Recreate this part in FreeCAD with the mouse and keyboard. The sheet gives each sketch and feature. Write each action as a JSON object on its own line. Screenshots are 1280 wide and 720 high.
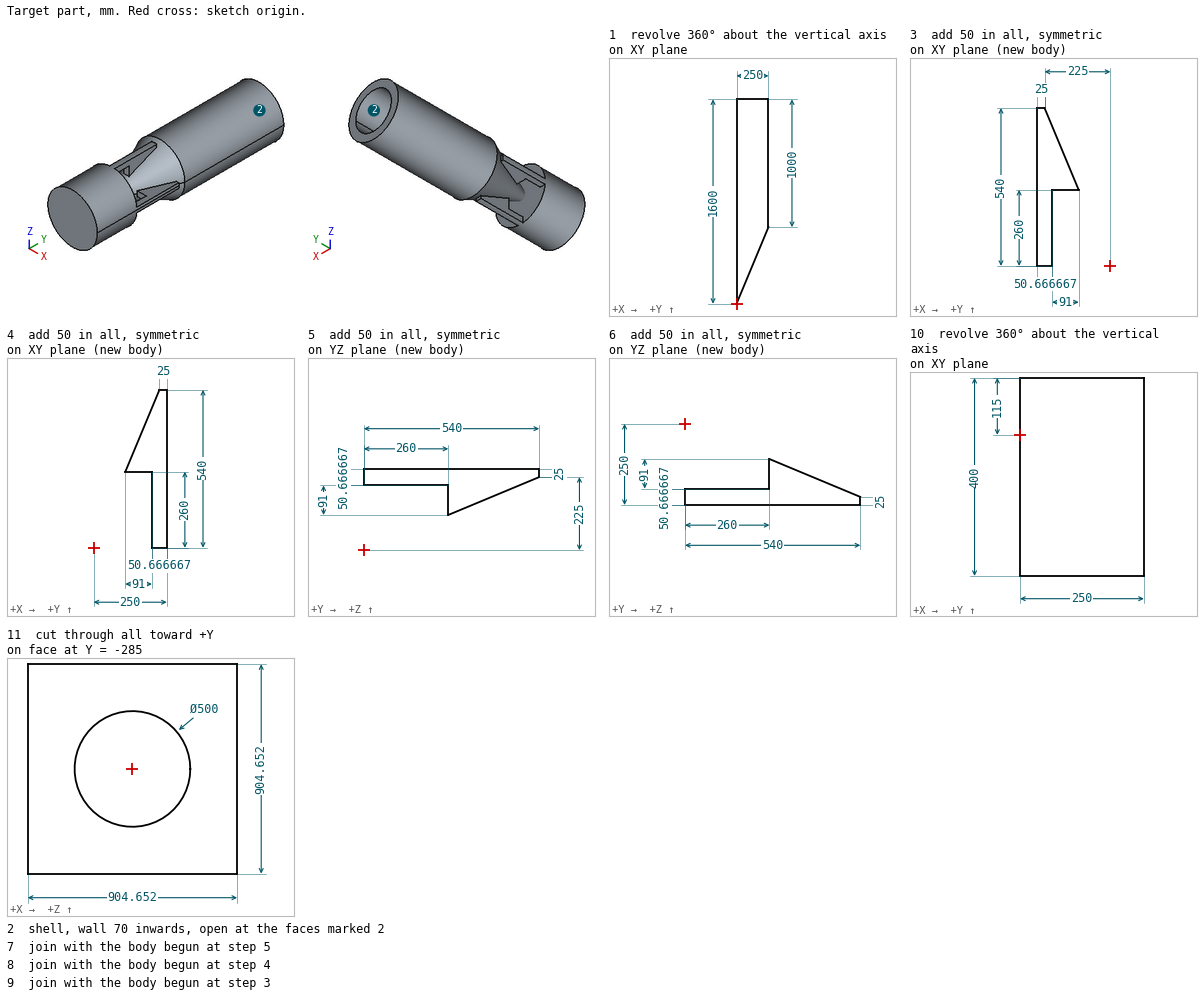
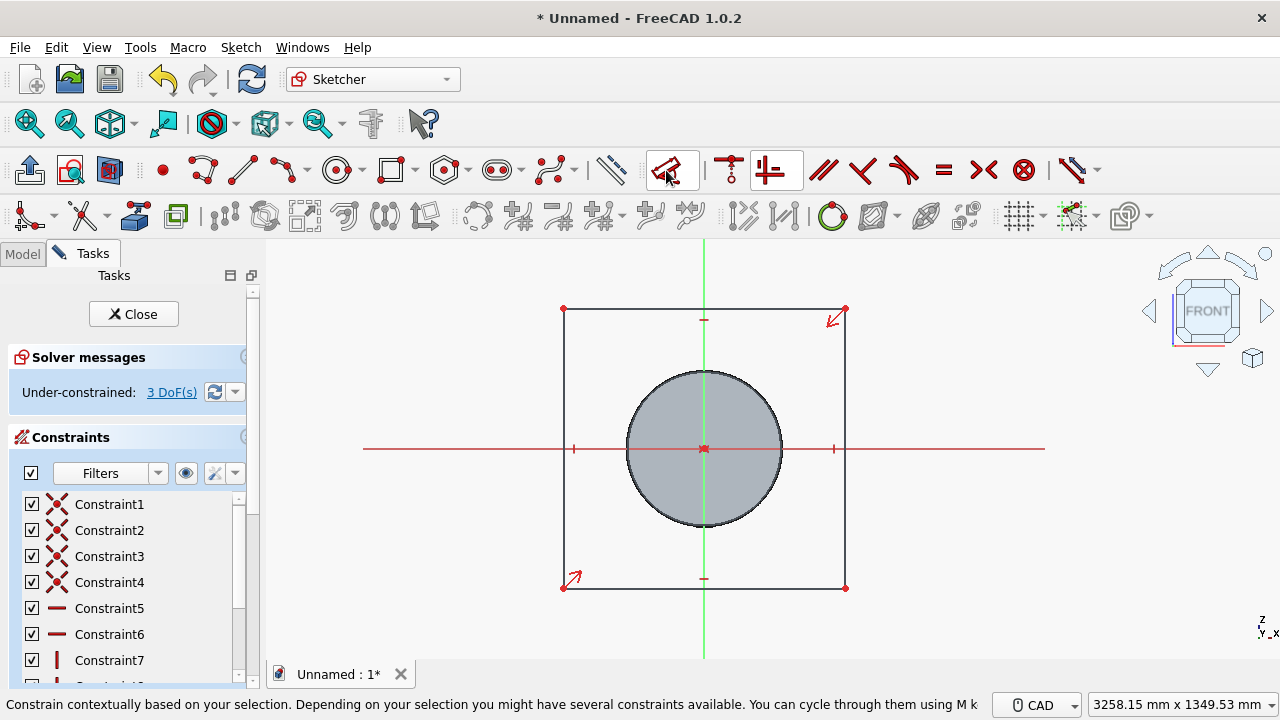
{"action": "left_click", "coordinate": [758, 394]}
{"action": "left_click", "coordinate": [780, 371]}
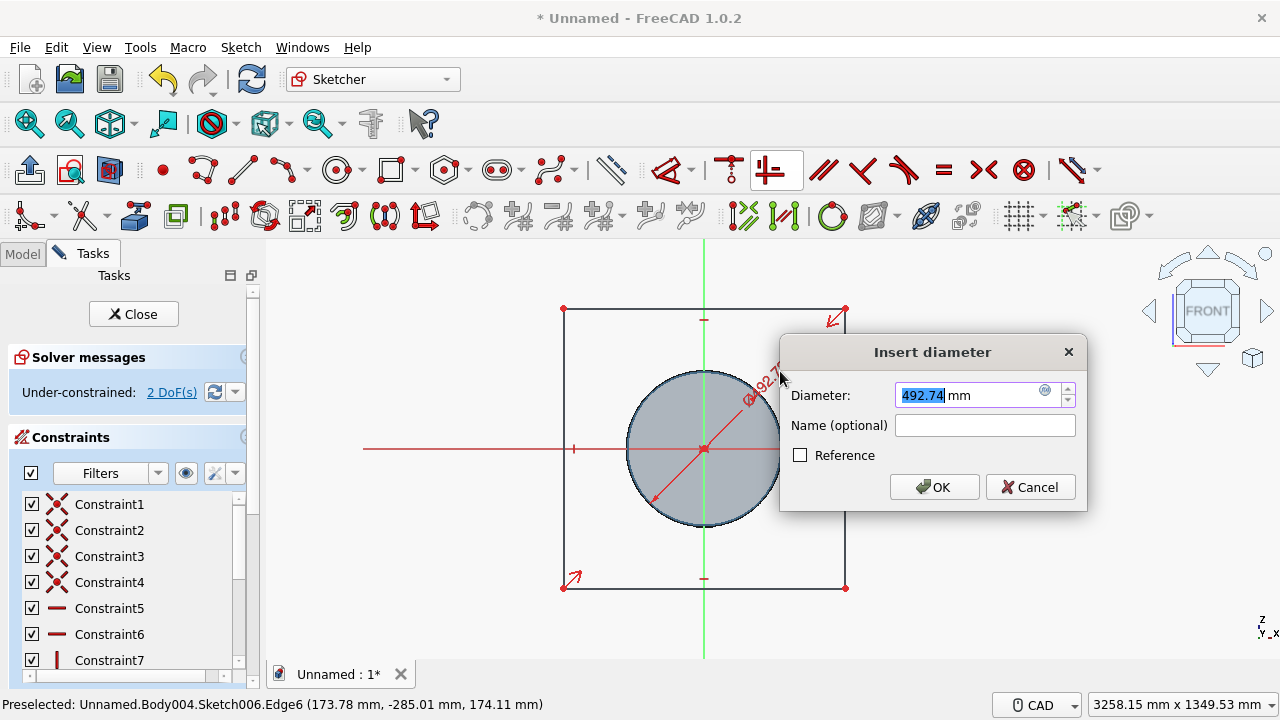
{"action": "type", "text": "500"}
{"action": "key", "text": "Return"}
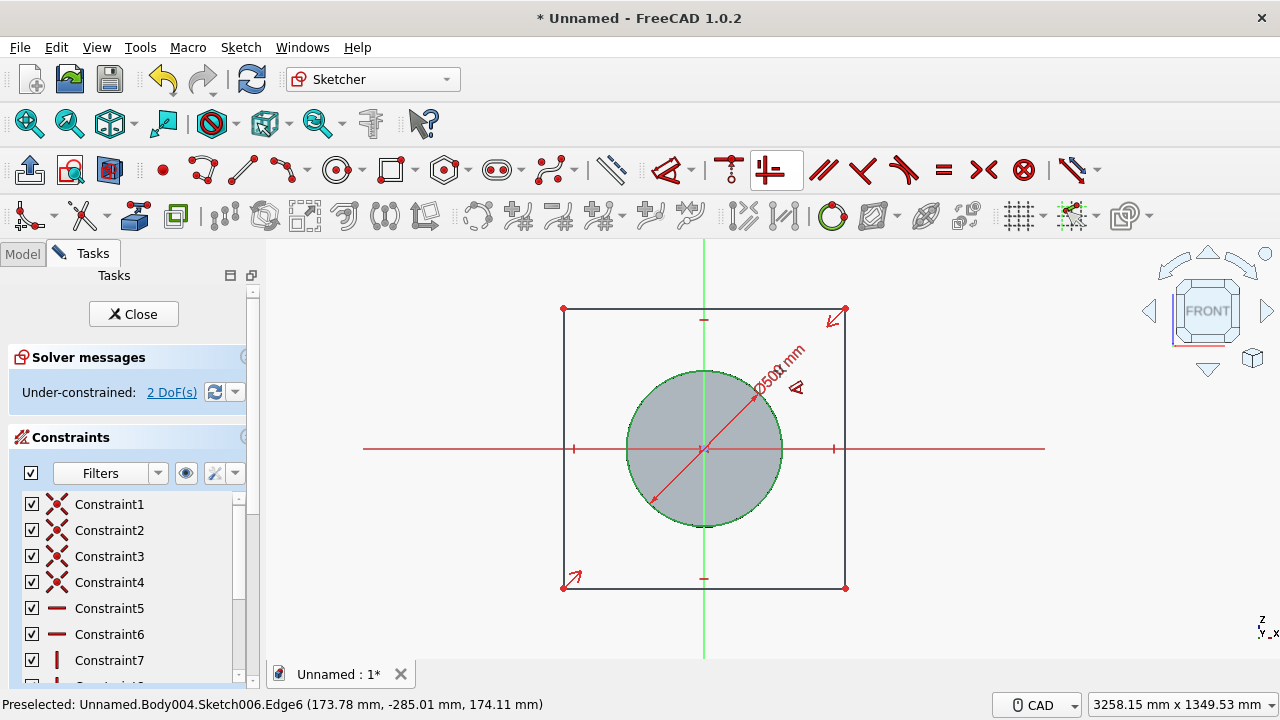
{"action": "left_click", "coordinate": [648, 589]}
{"action": "left_click", "coordinate": [640, 623]}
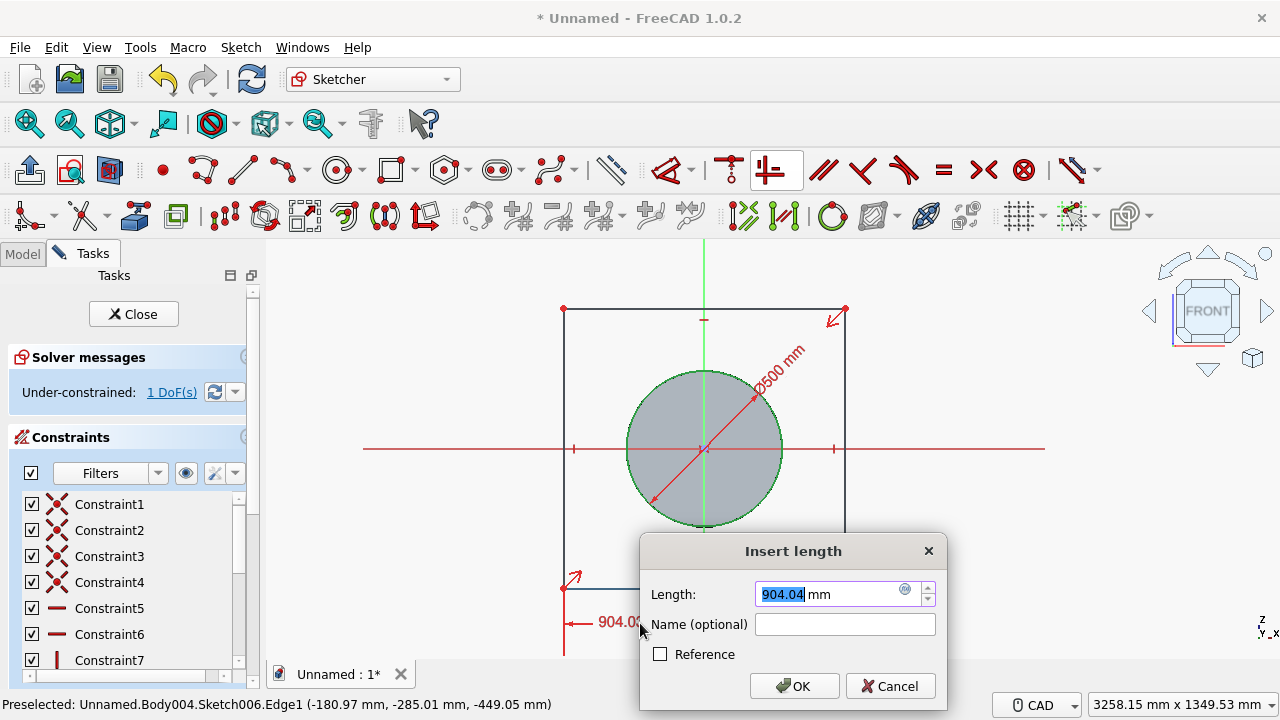
{"action": "type", "text": "904.652"}
{"action": "key", "text": "Return"}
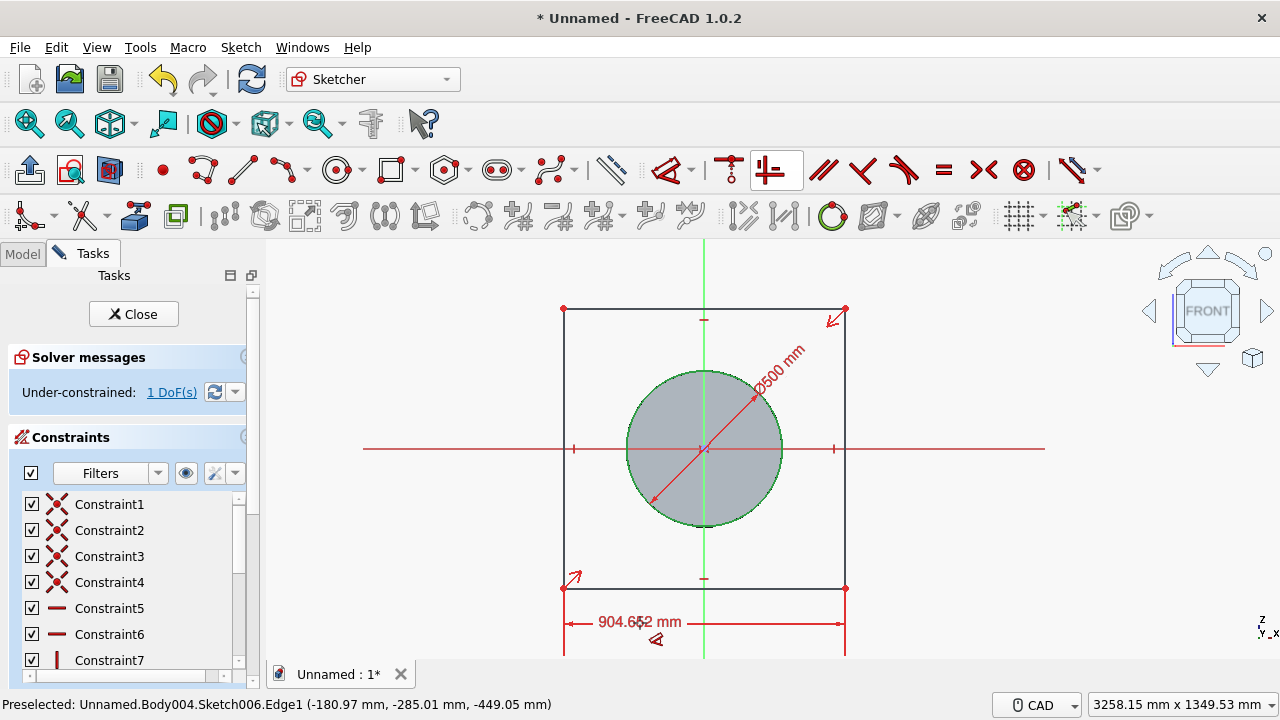
{"action": "left_click", "coordinate": [845, 505]}
{"action": "left_click", "coordinate": [879, 384]}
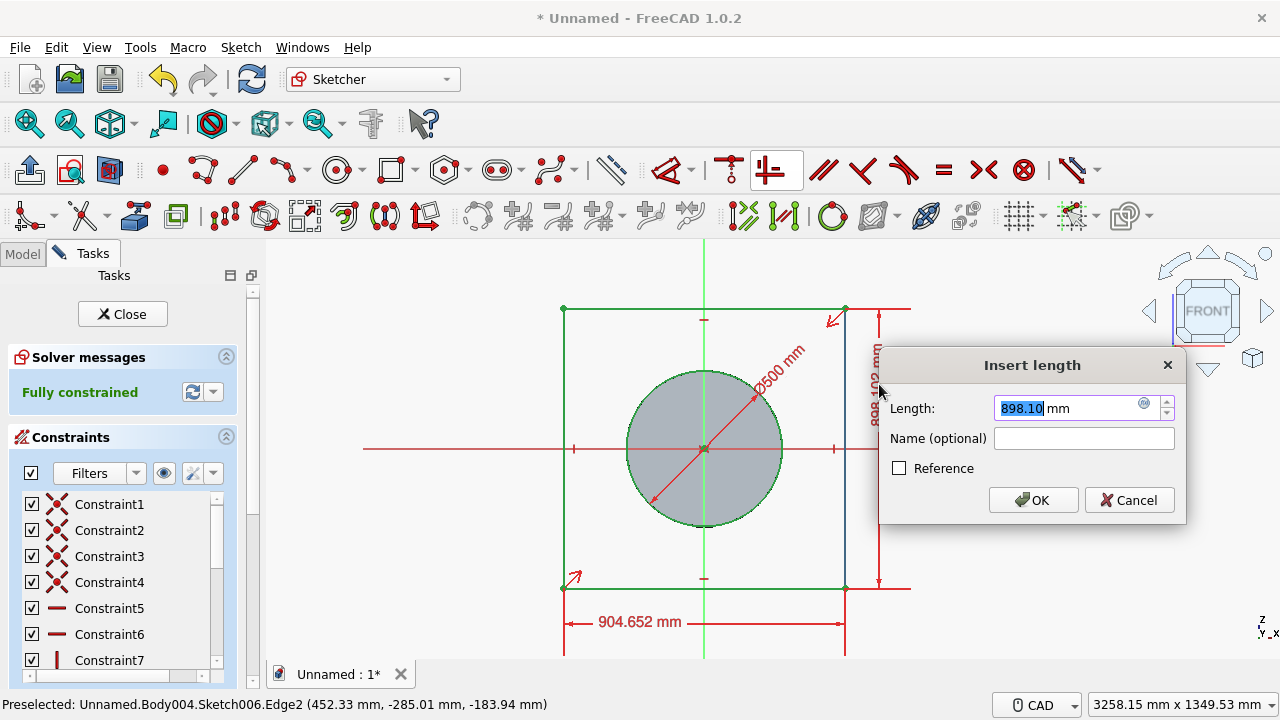
{"action": "type", "text": "904.652"}
{"action": "key", "text": "Return"}
{"action": "key", "text": "Escape"}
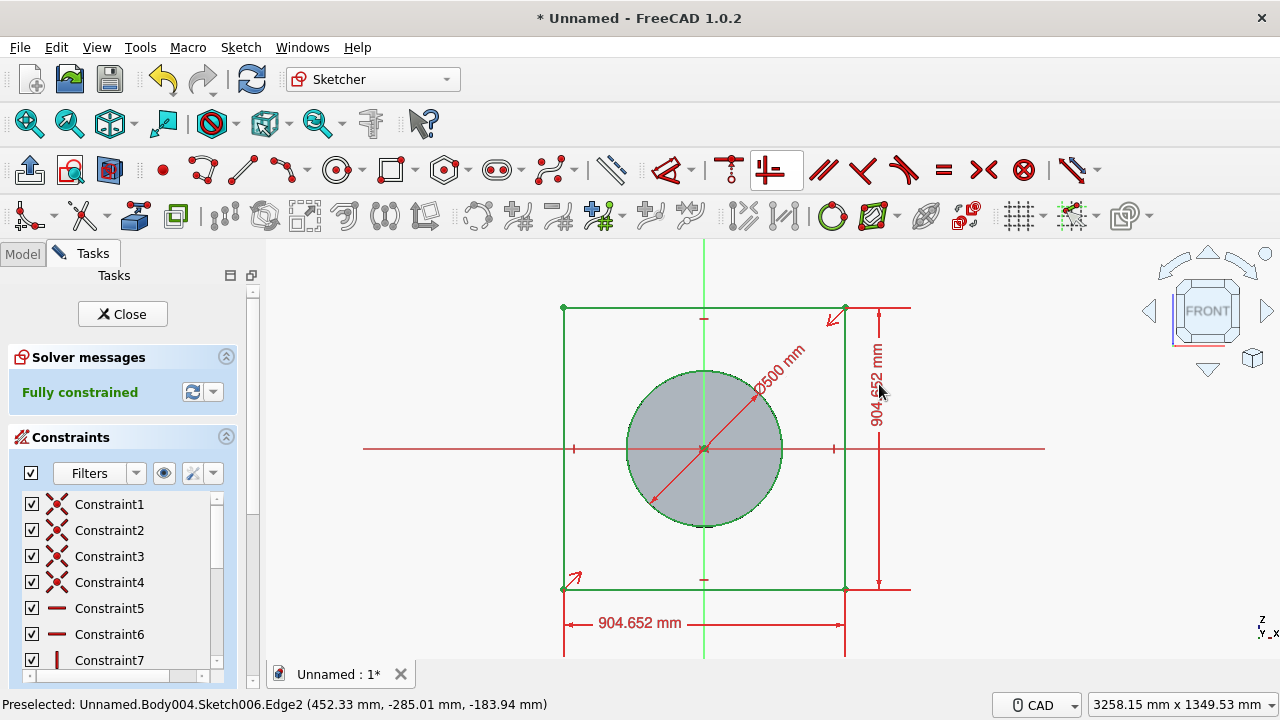
{"action": "left_click", "coordinate": [123, 314]}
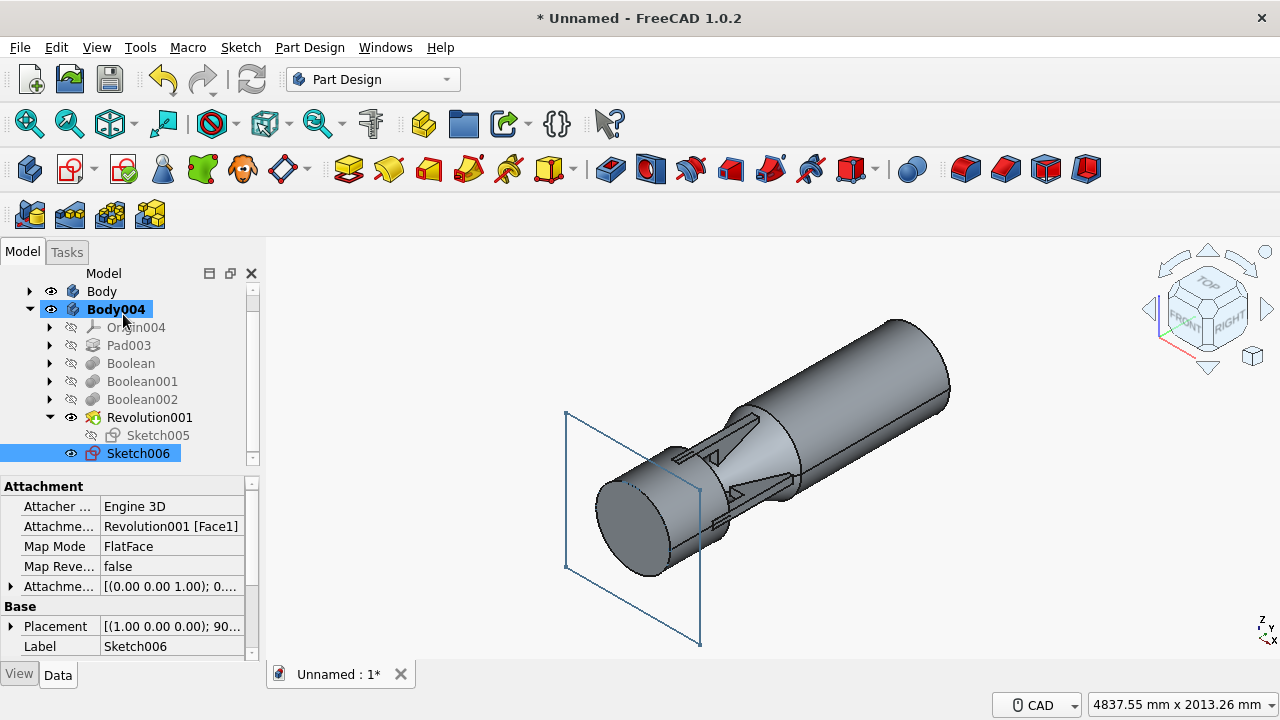
{"action": "left_click", "coordinate": [612, 170]}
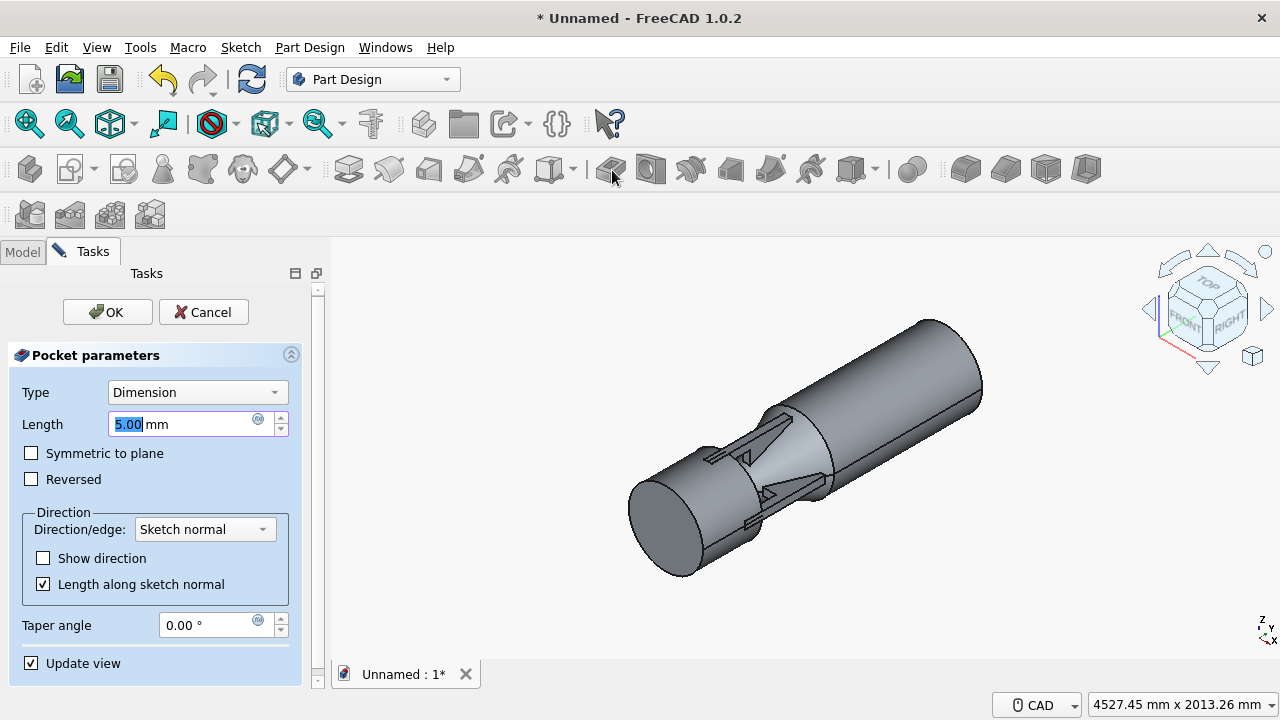
{"action": "left_click", "coordinate": [198, 392]}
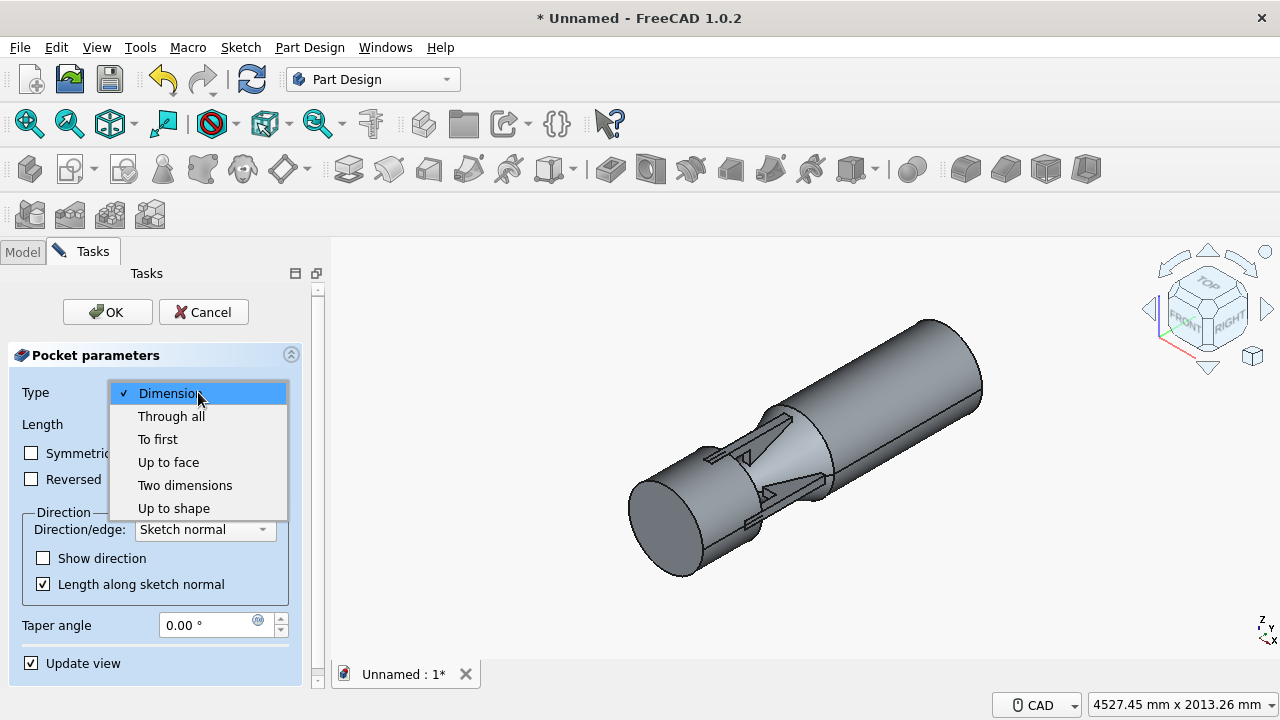
{"action": "left_click", "coordinate": [198, 416]}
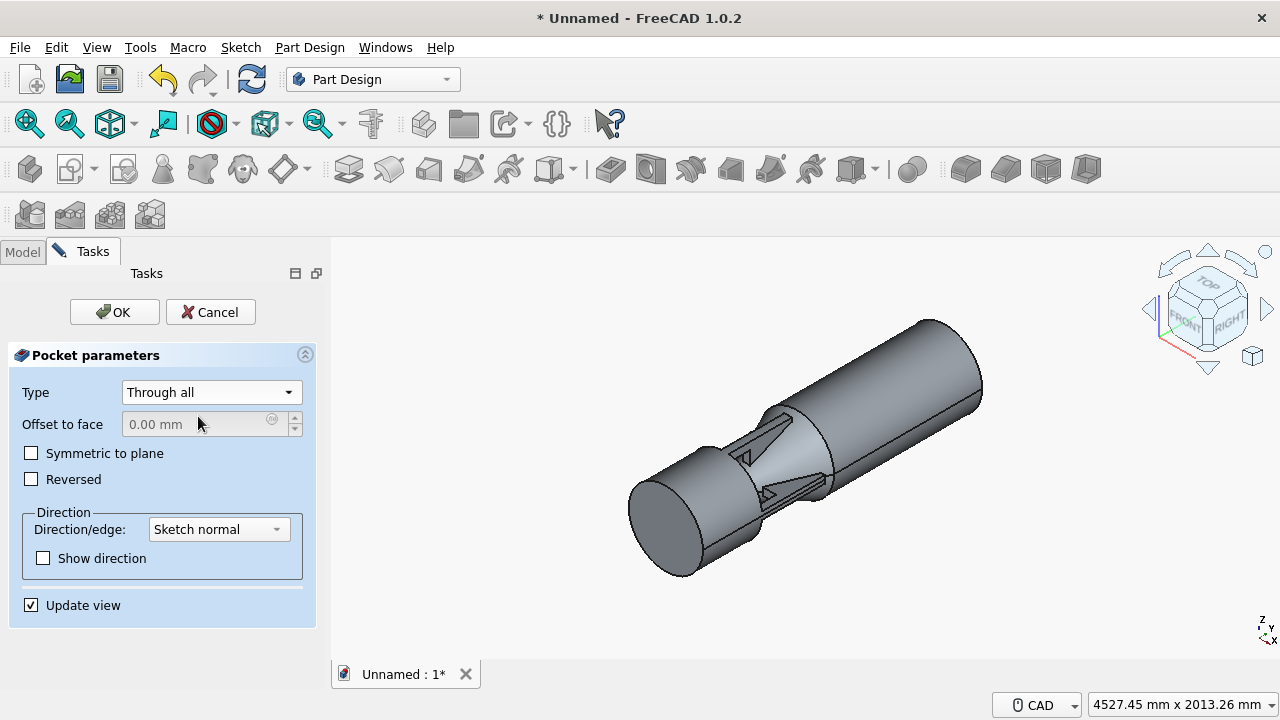
{"action": "left_click", "coordinate": [115, 312]}